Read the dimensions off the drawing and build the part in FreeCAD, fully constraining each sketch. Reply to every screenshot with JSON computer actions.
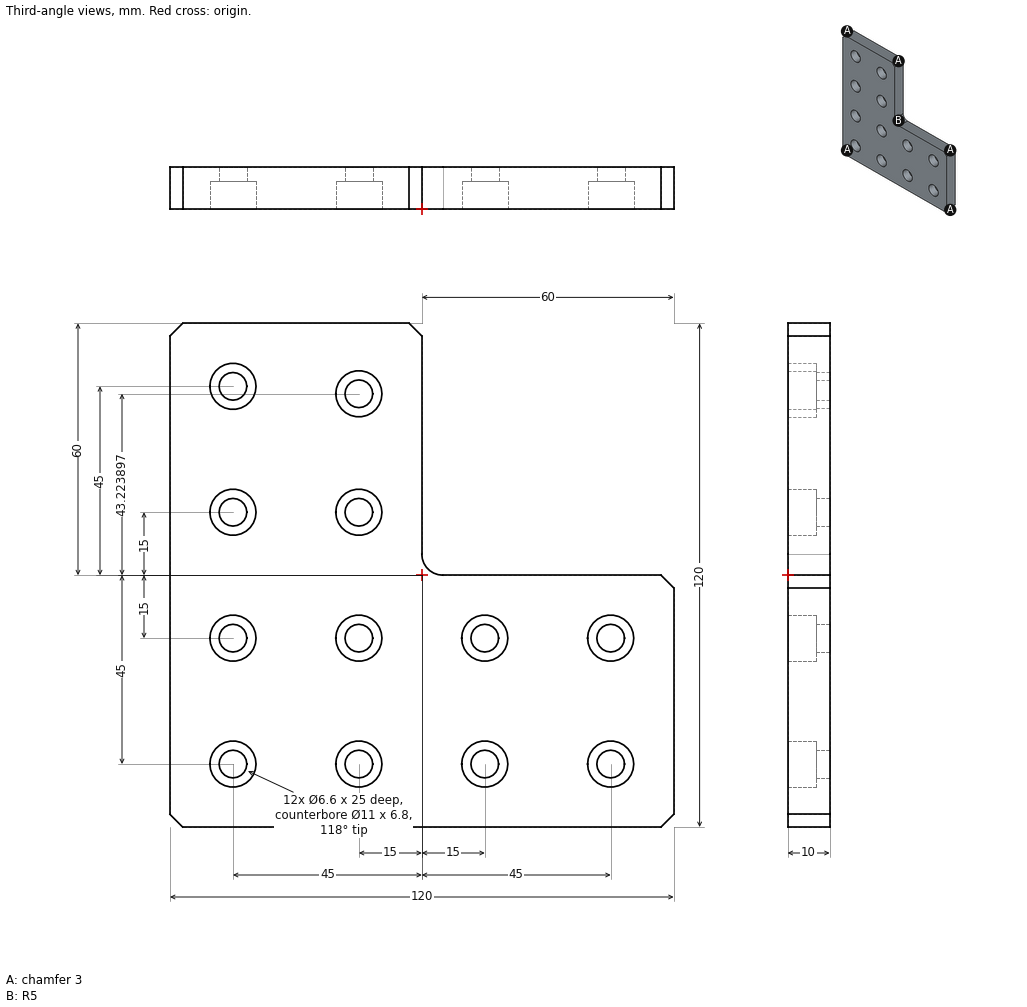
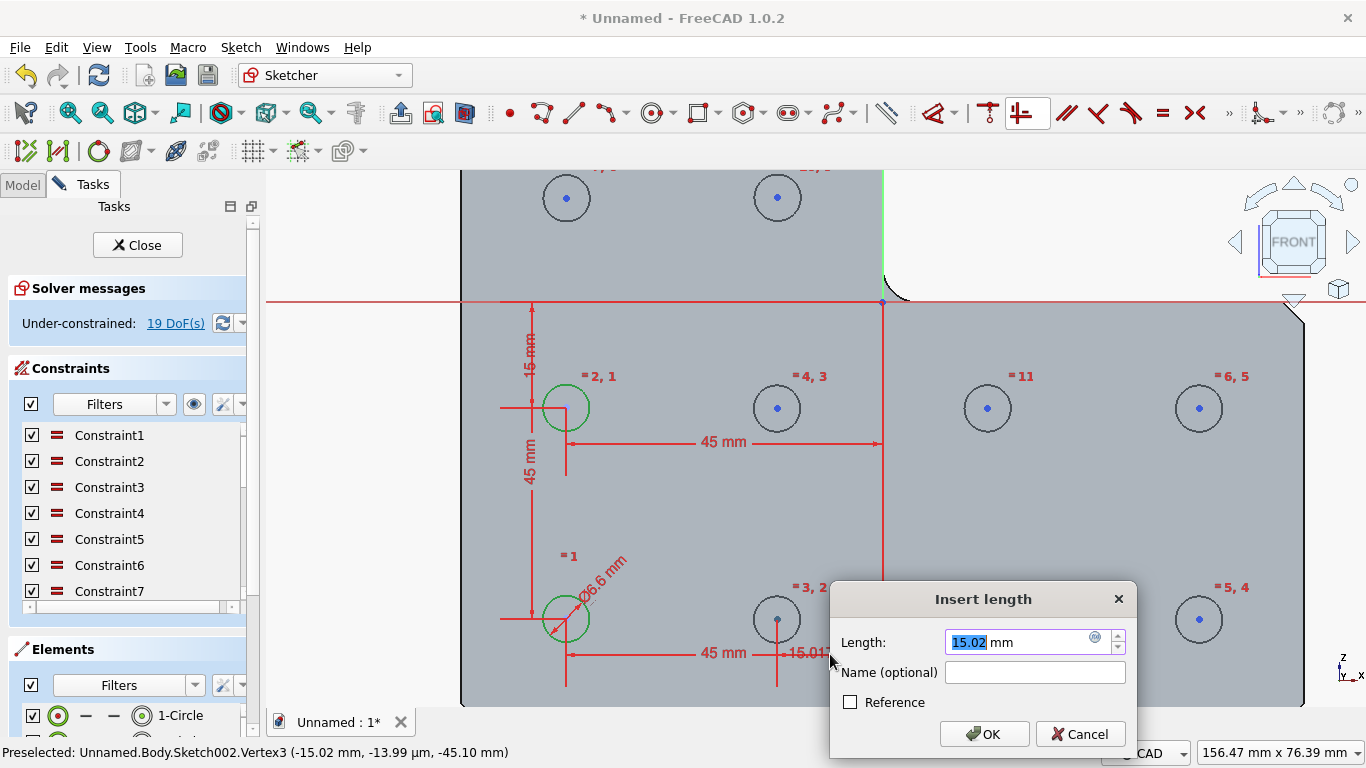
{"action": "type", "text": "15"}
{"action": "key", "text": "Return"}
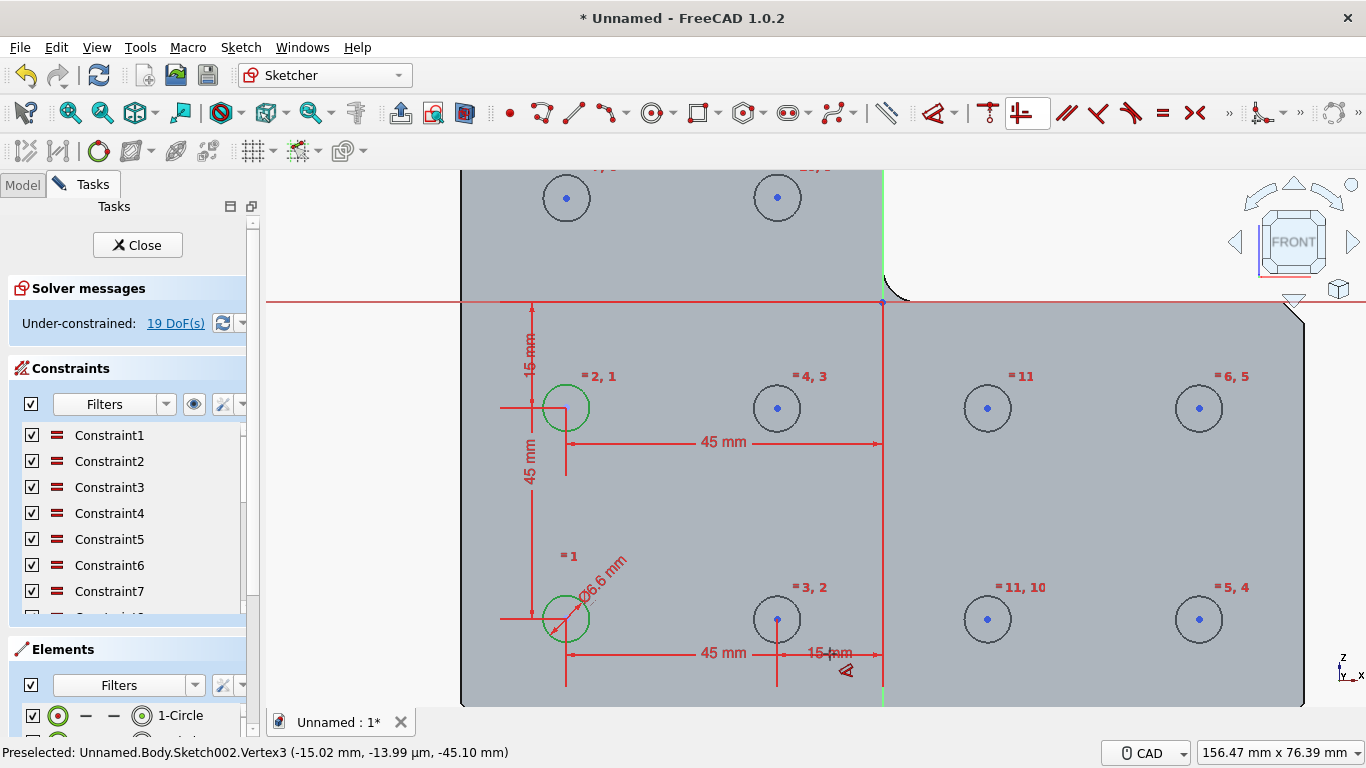
{"action": "left_click", "coordinate": [777, 620]}
{"action": "left_click", "coordinate": [743, 388]}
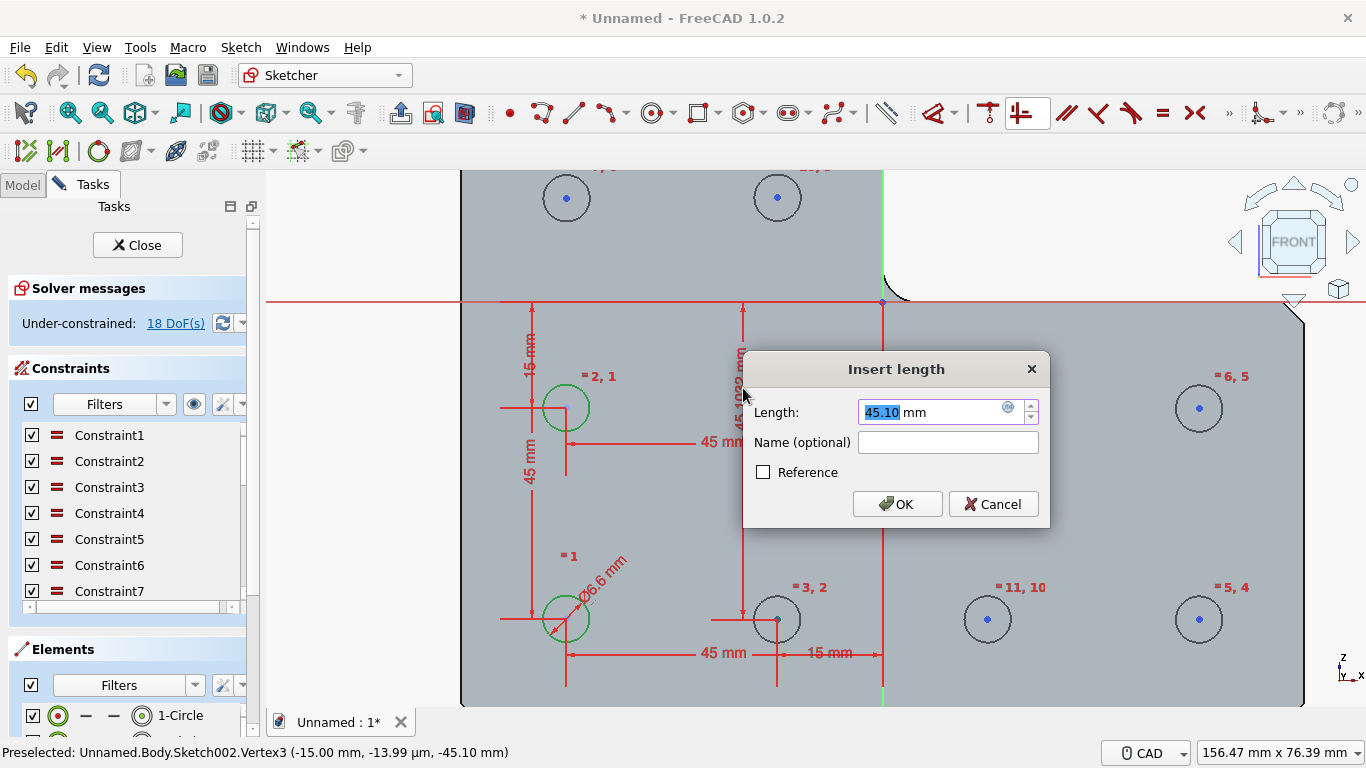
{"action": "type", "text": "45"}
{"action": "key", "text": "Return"}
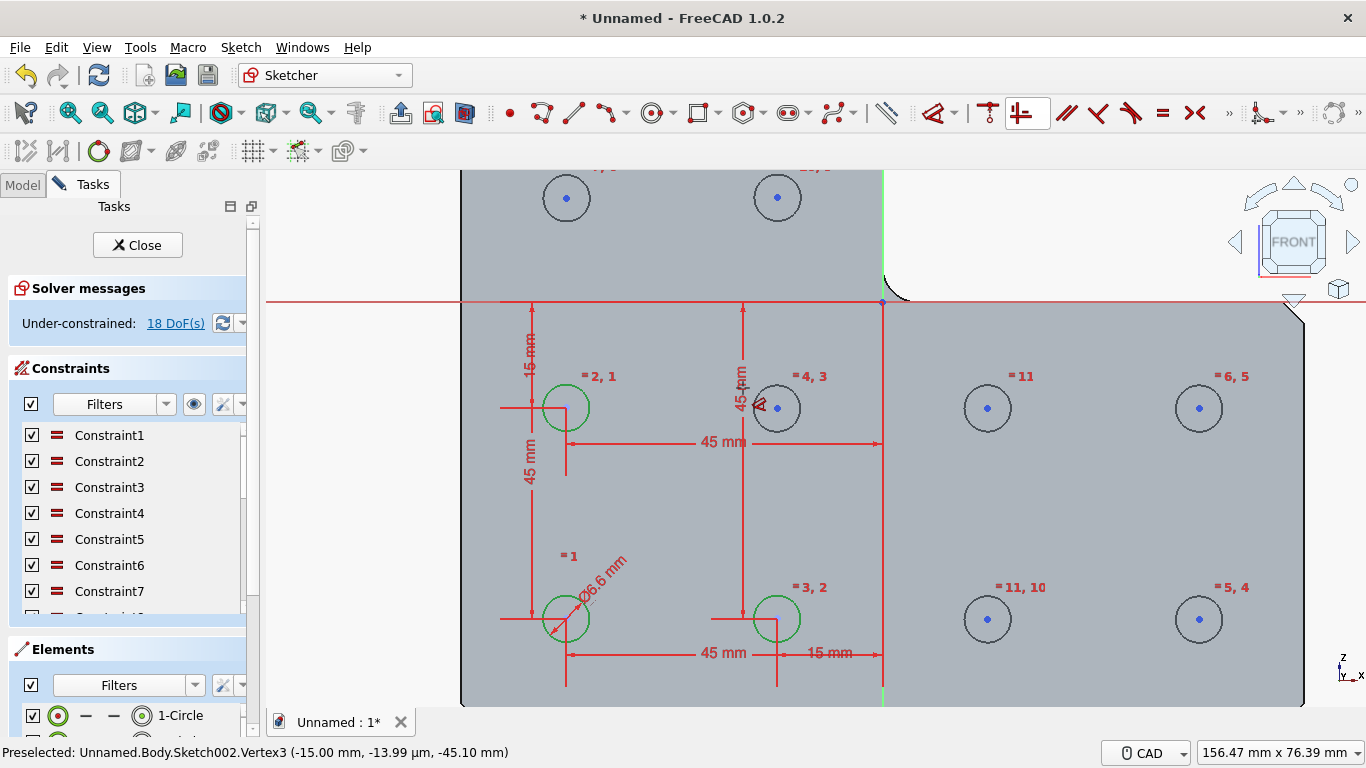
{"action": "left_click", "coordinate": [777, 409]}
{"action": "left_click", "coordinate": [830, 443]}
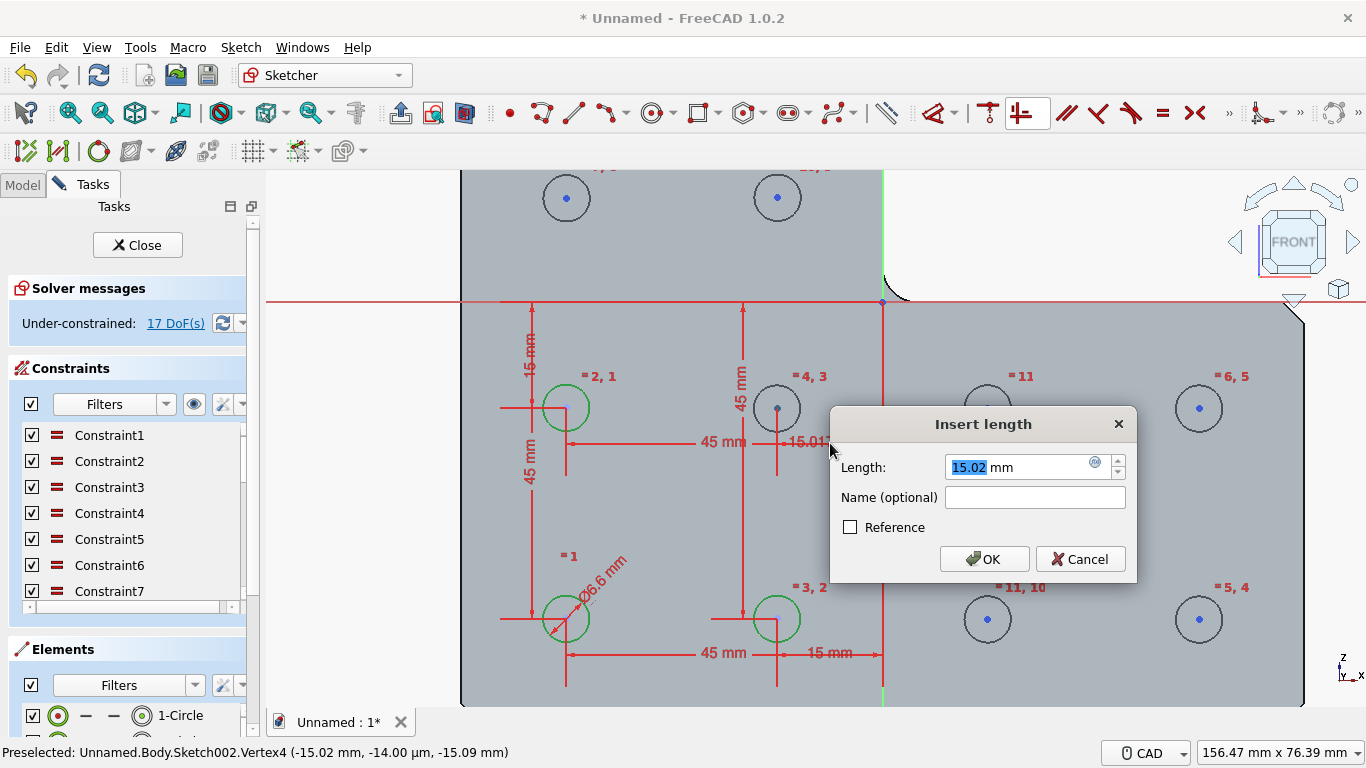
{"action": "type", "text": "15"}
{"action": "key", "text": "Return"}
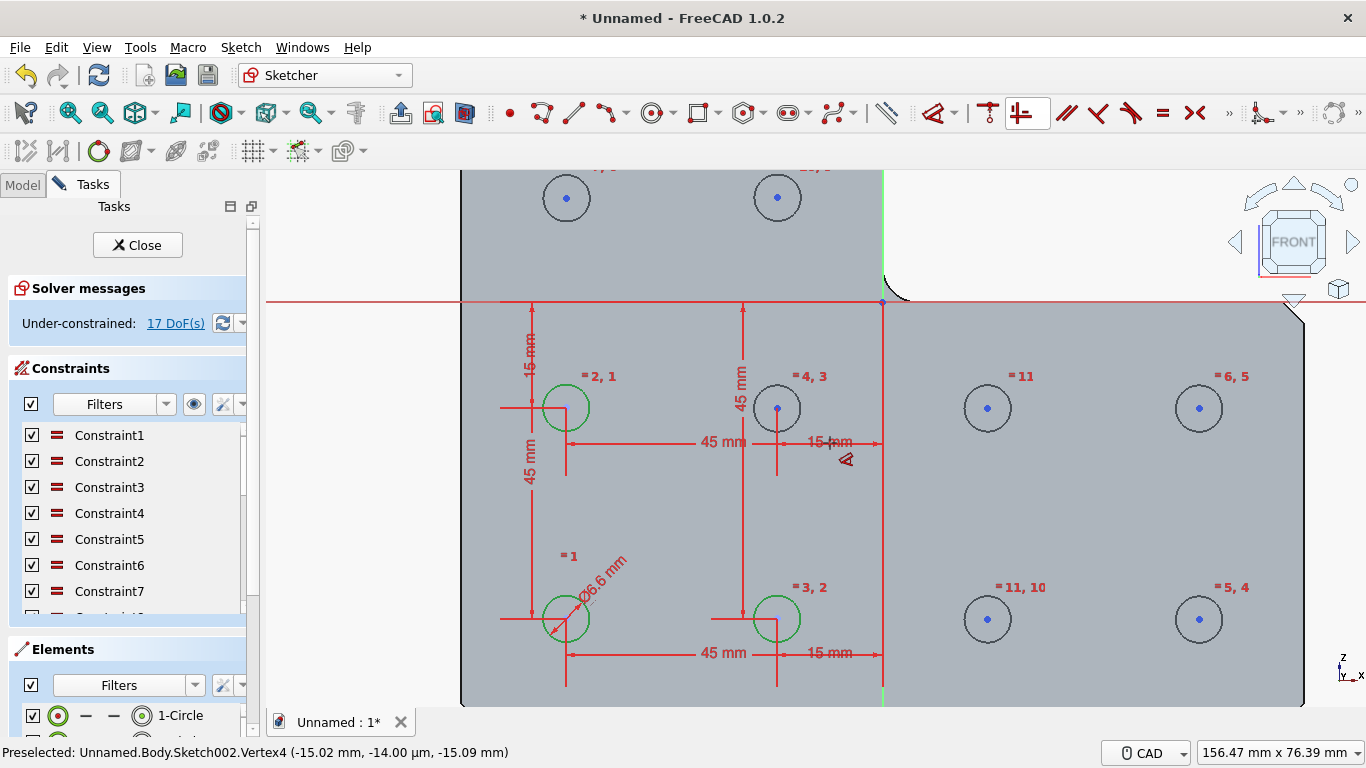
{"action": "left_click", "coordinate": [777, 409]}
{"action": "left_click", "coordinate": [743, 355]}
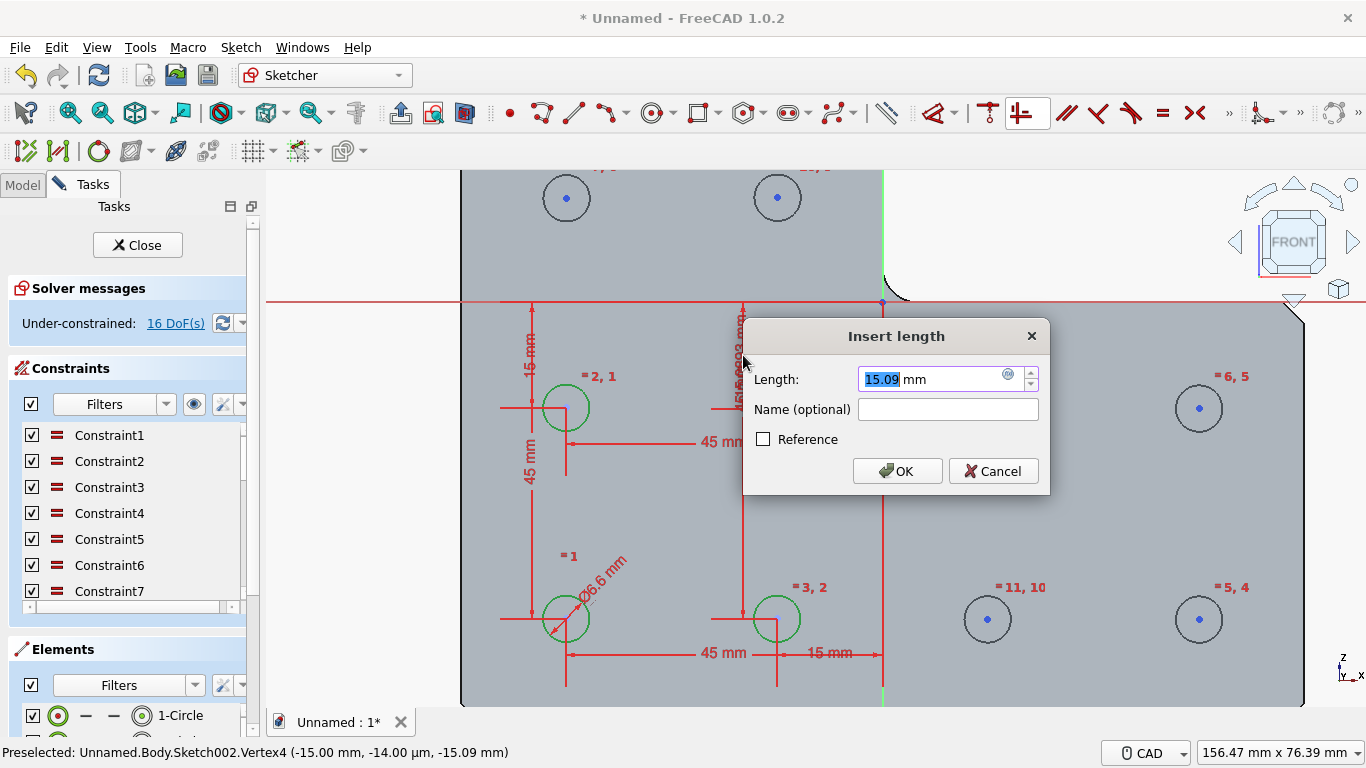
{"action": "type", "text": "15"}
{"action": "key", "text": "Return"}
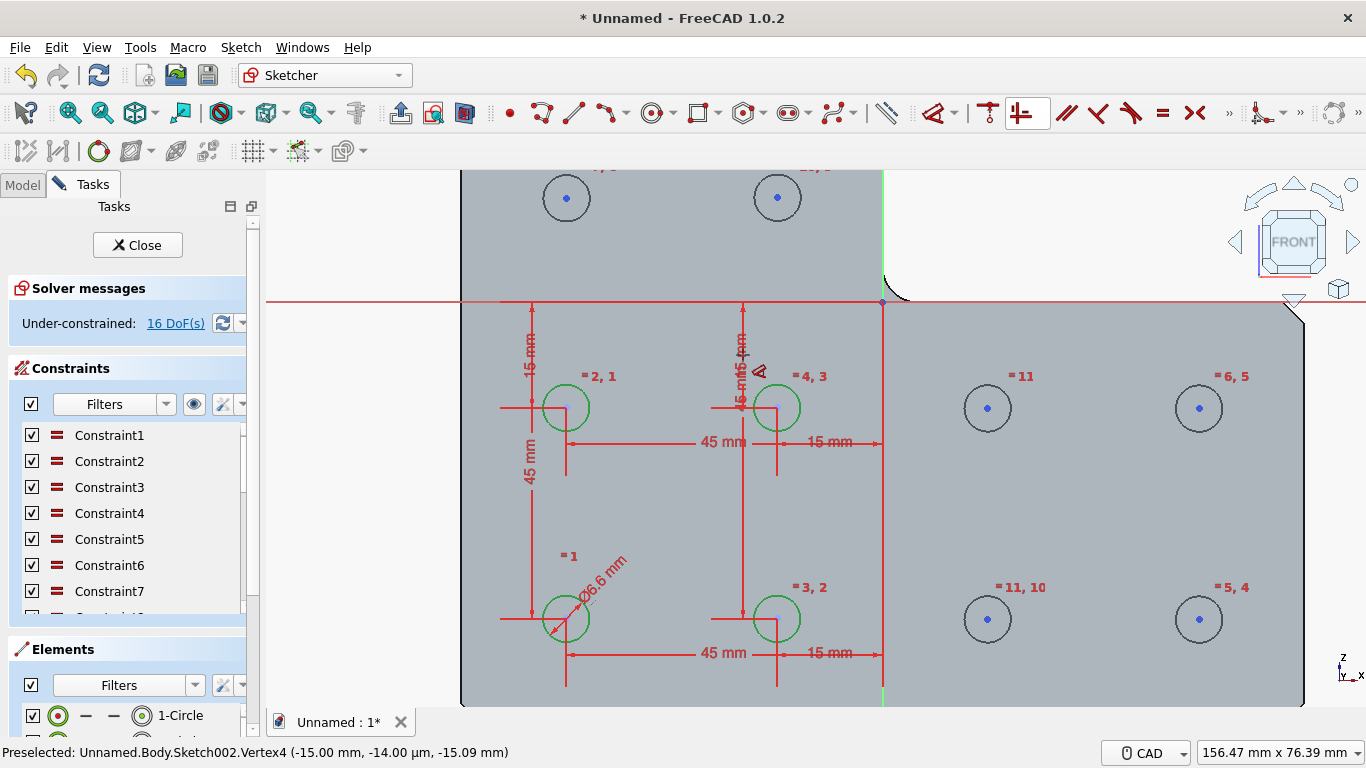
{"action": "left_click", "coordinate": [1199, 620]}
{"action": "left_click", "coordinate": [1041, 654]}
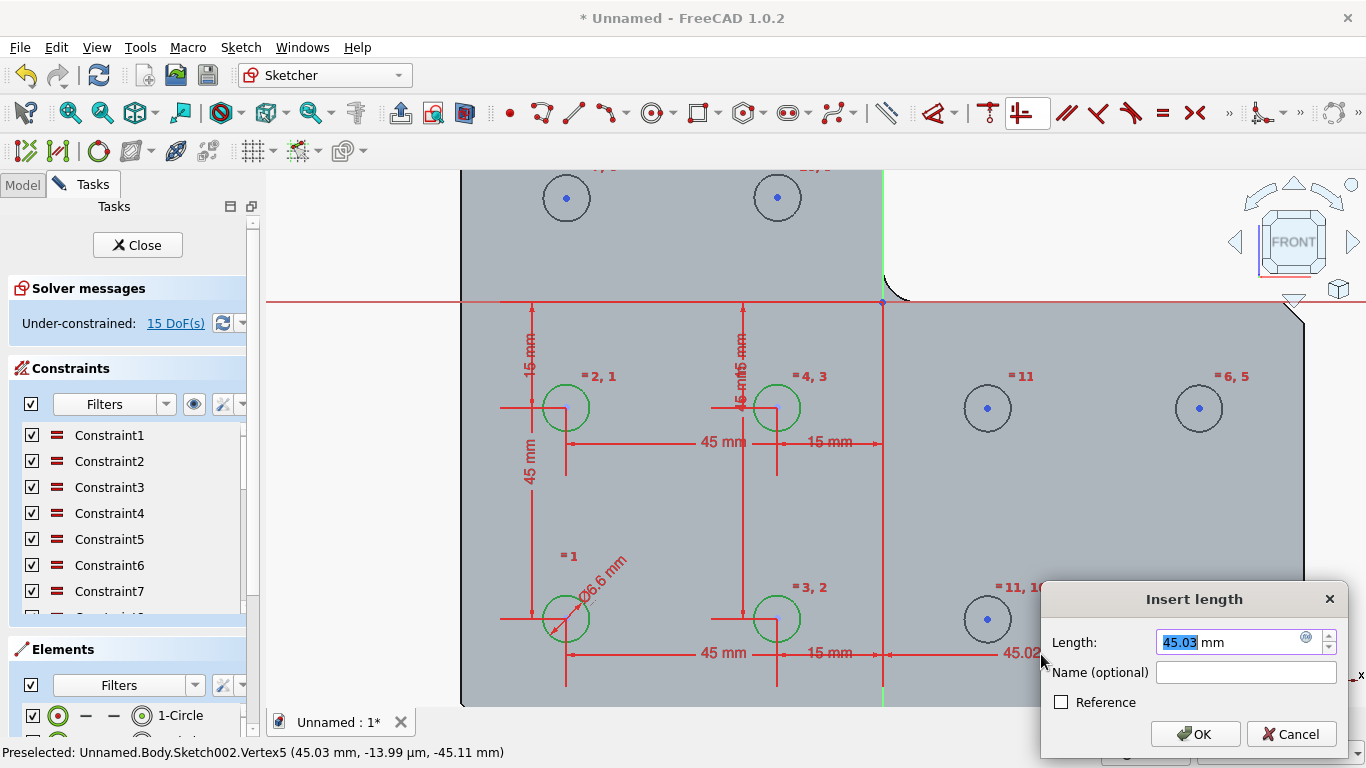
{"action": "type", "text": "45"}
{"action": "key", "text": "Return"}